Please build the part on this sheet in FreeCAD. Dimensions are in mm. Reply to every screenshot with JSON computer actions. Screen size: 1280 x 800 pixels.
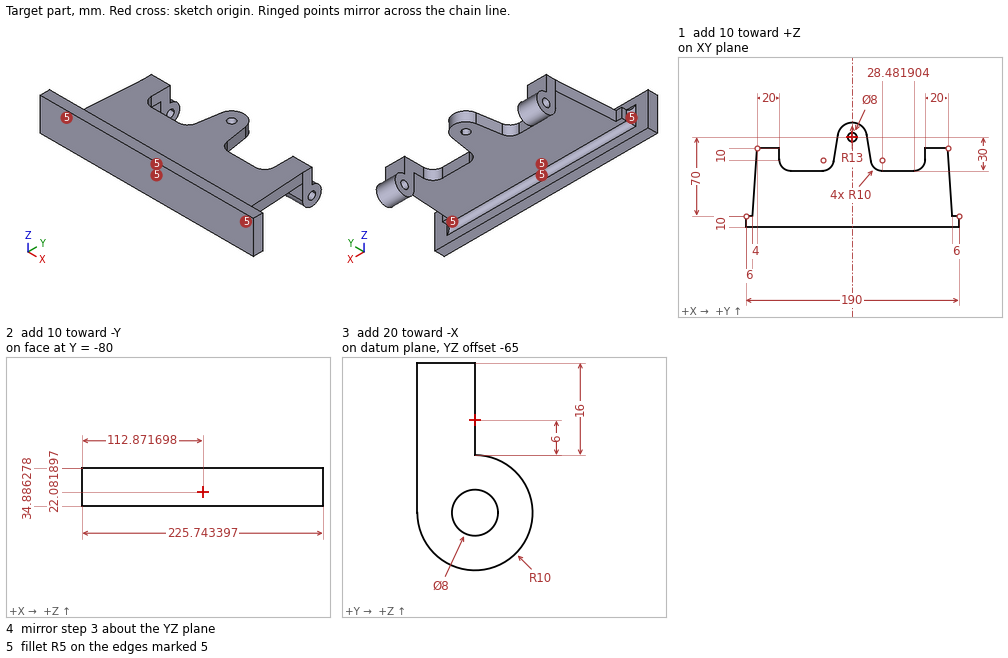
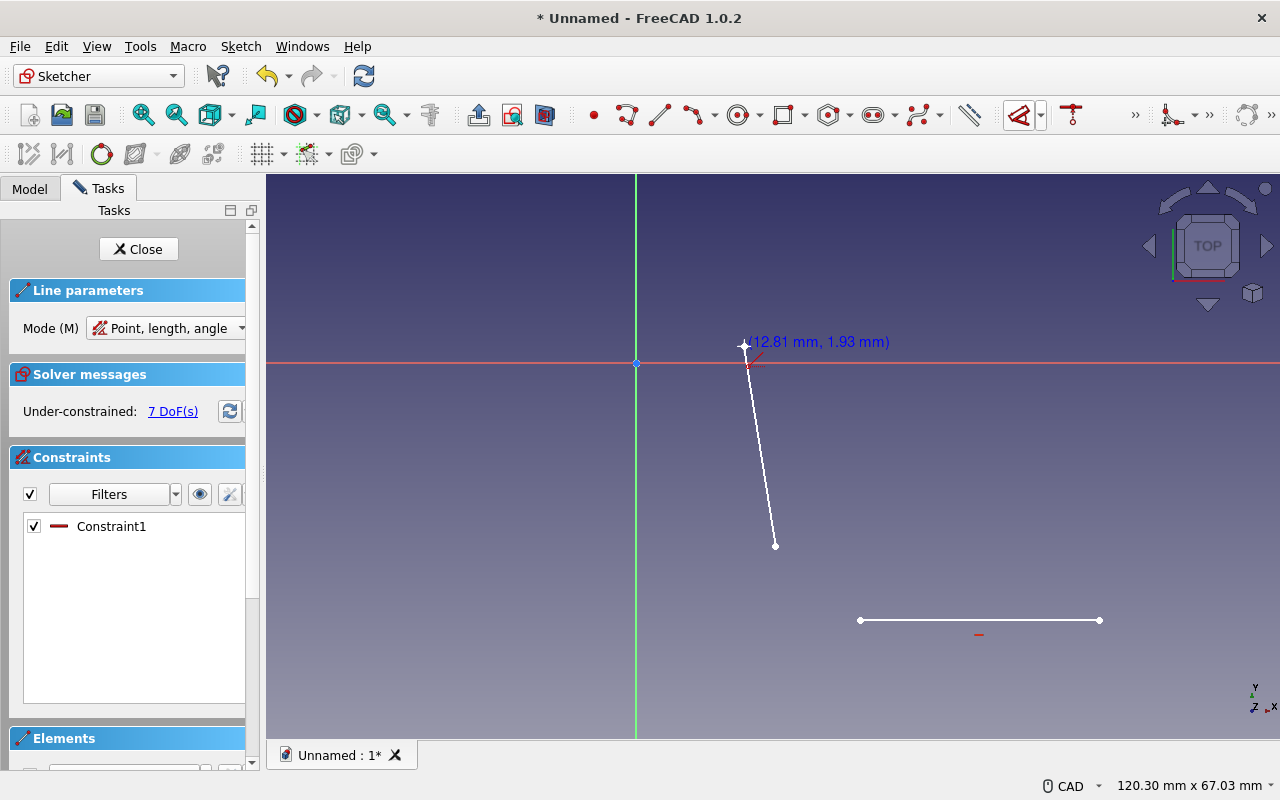
{"action": "left_click", "coordinate": [528, 346]}
{"action": "left_click", "coordinate": [496, 545]}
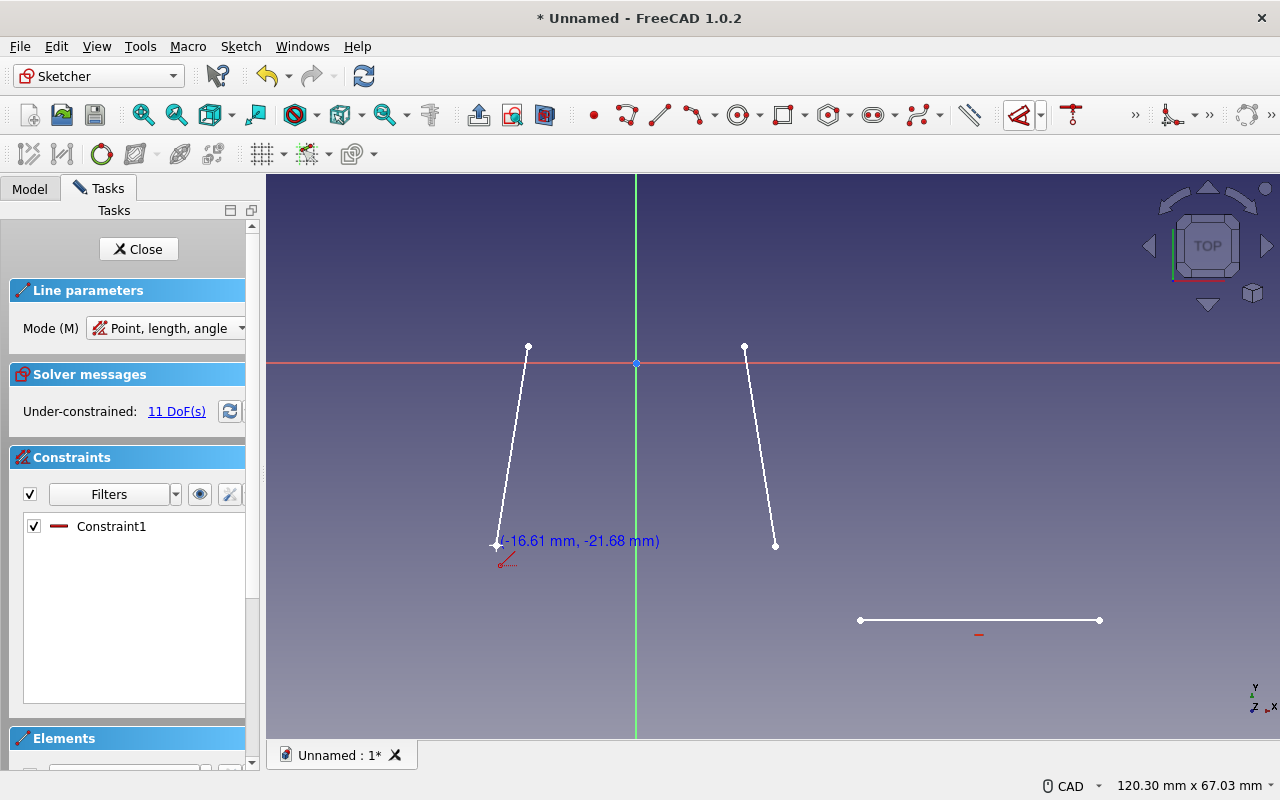
{"action": "left_click", "coordinate": [413, 616]}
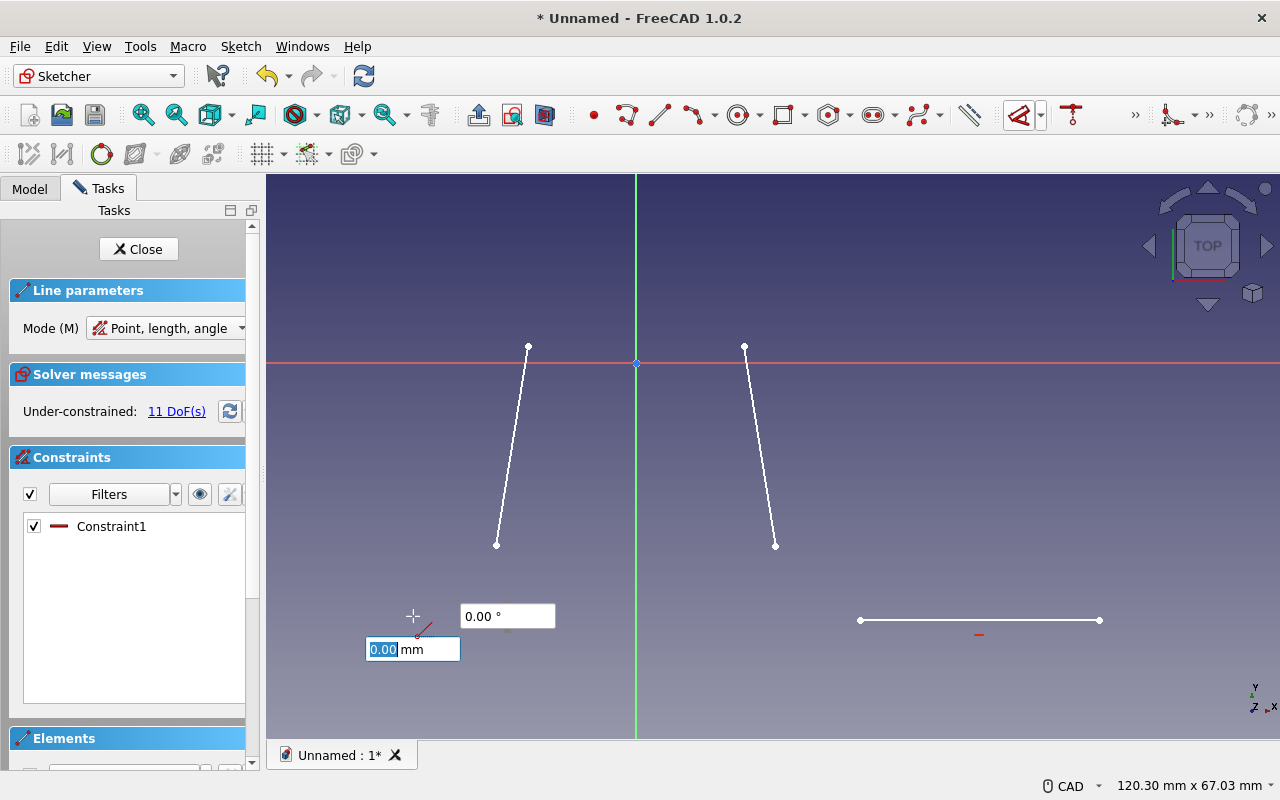
{"action": "scroll", "coordinate": [744, 346], "scroll_direction": "down", "scroll_amount": 5}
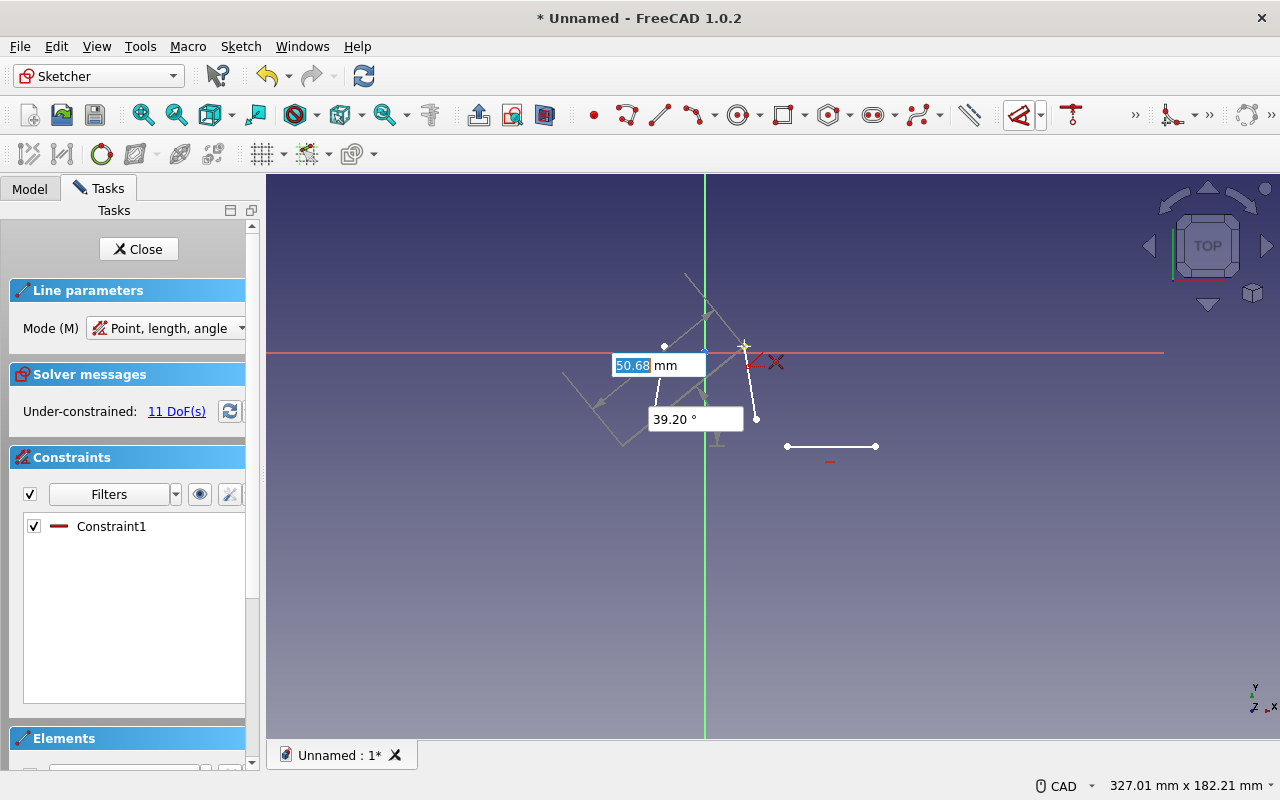
{"action": "left_click", "coordinate": [534, 446]}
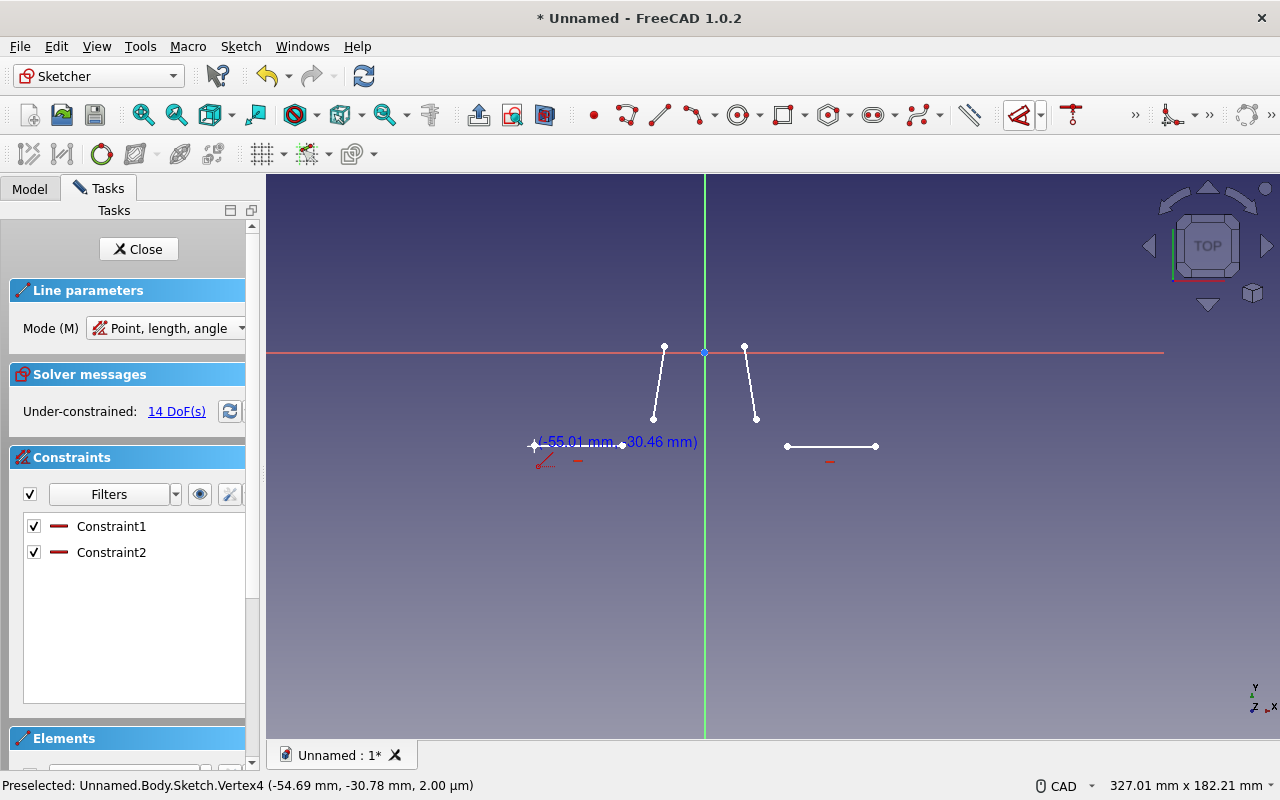
{"action": "left_click", "coordinate": [627, 116]}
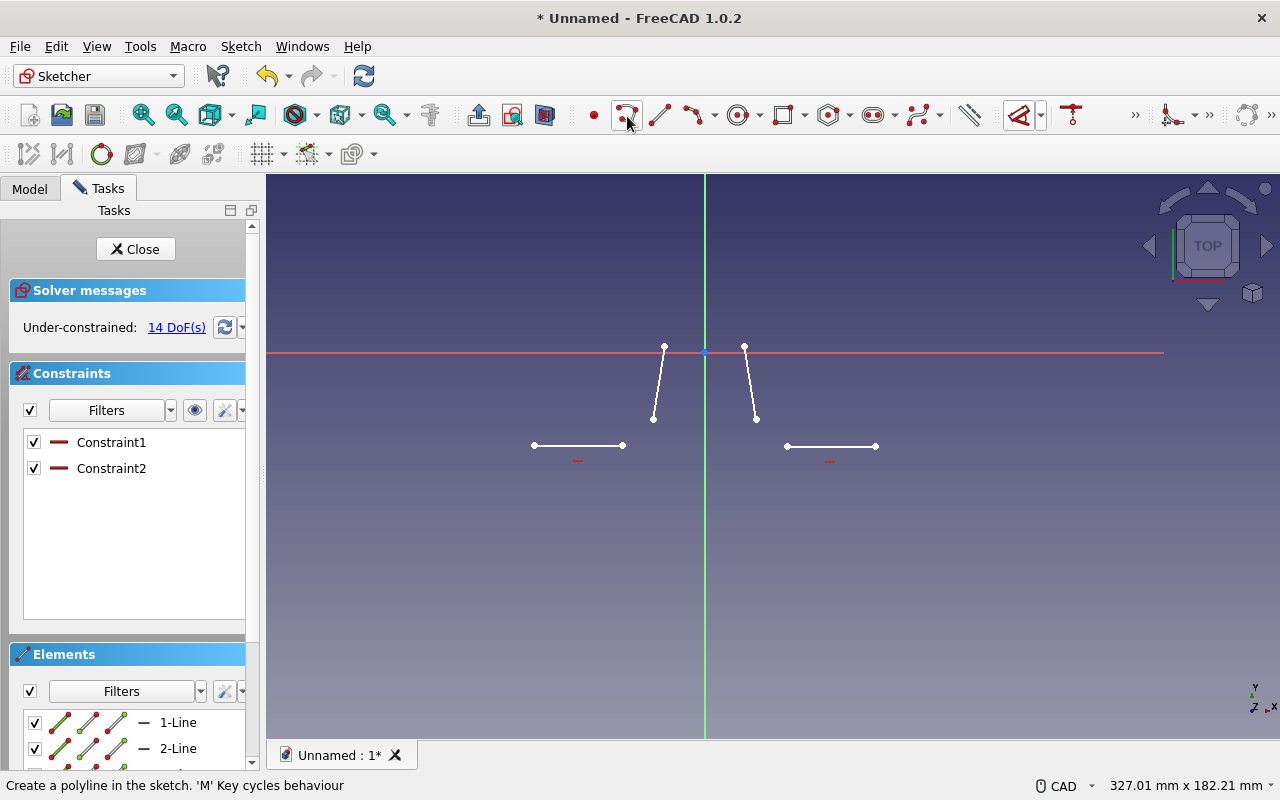
{"action": "left_click", "coordinate": [503, 415]}
{"action": "left_click", "coordinate": [503, 384]}
{"action": "left_click", "coordinate": [441, 384]}
{"action": "left_click", "coordinate": [429, 570]}
{"action": "left_click", "coordinate": [410, 570]}
{"action": "left_click", "coordinate": [410, 601]}
{"action": "left_click", "coordinate": [999, 601]}
{"action": "left_click", "coordinate": [999, 570]}
{"action": "left_click", "coordinate": [981, 570]}
{"action": "left_click", "coordinate": [968, 384]}
{"action": "left_click", "coordinate": [906, 384]}
{"action": "left_click", "coordinate": [906, 415]}
{"action": "right_click", "coordinate": [906, 415]}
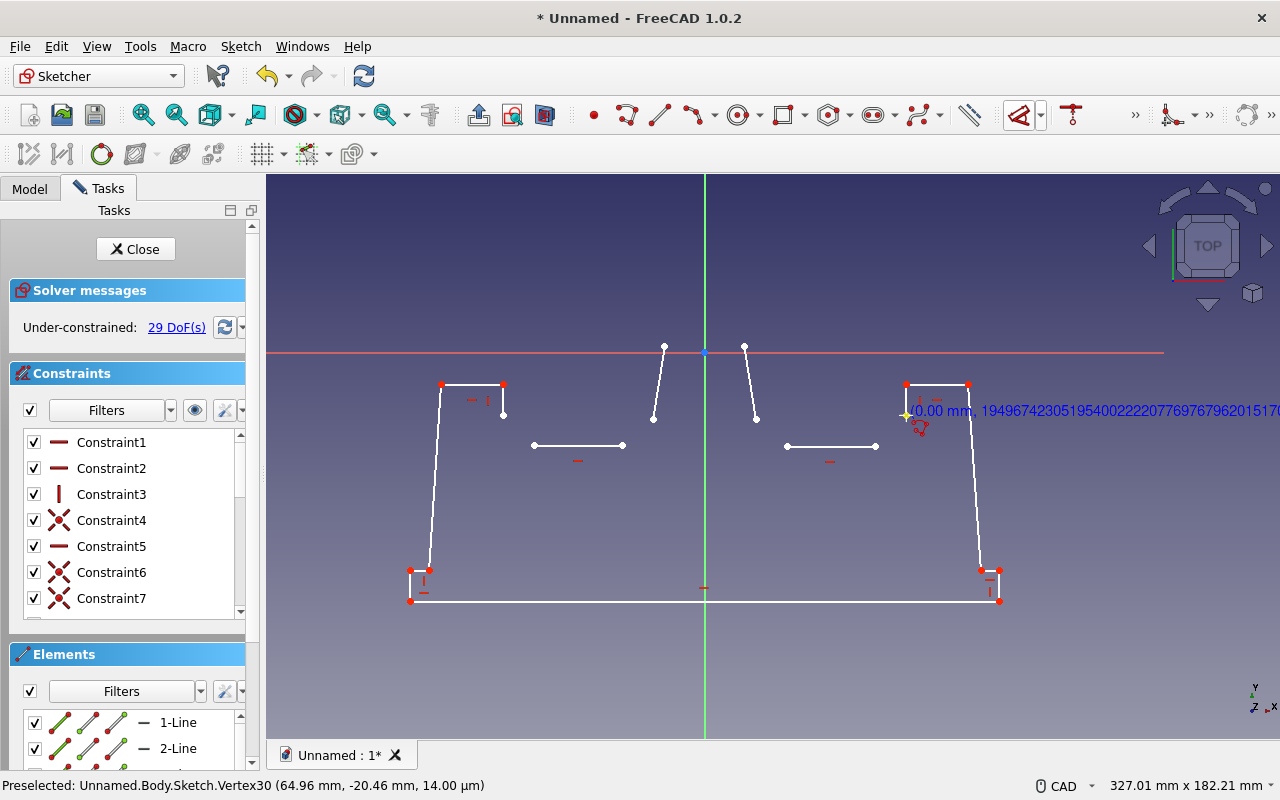
{"action": "left_click", "coordinate": [692, 116]}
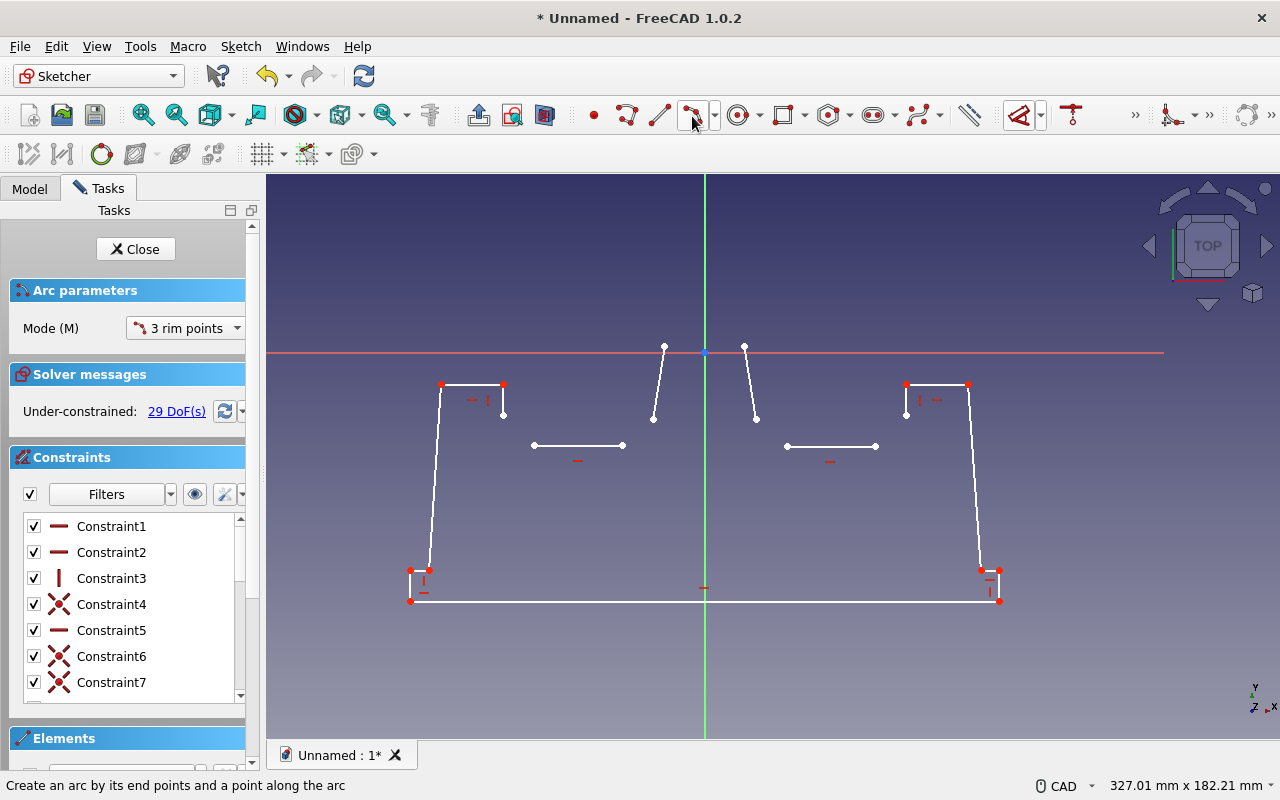
{"action": "left_click", "coordinate": [787, 447]}
{"action": "left_click", "coordinate": [756, 420]}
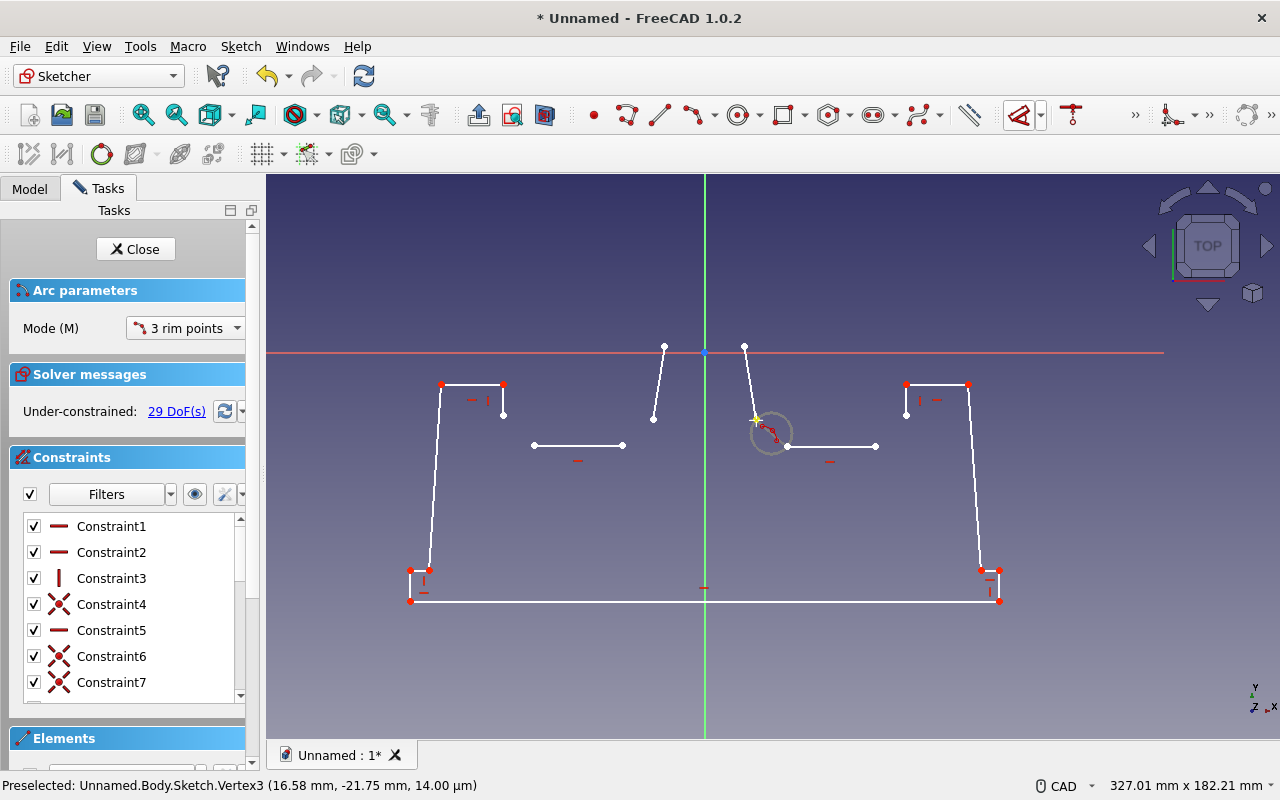
{"action": "scroll", "coordinate": [767, 438], "scroll_direction": "up", "scroll_amount": 4}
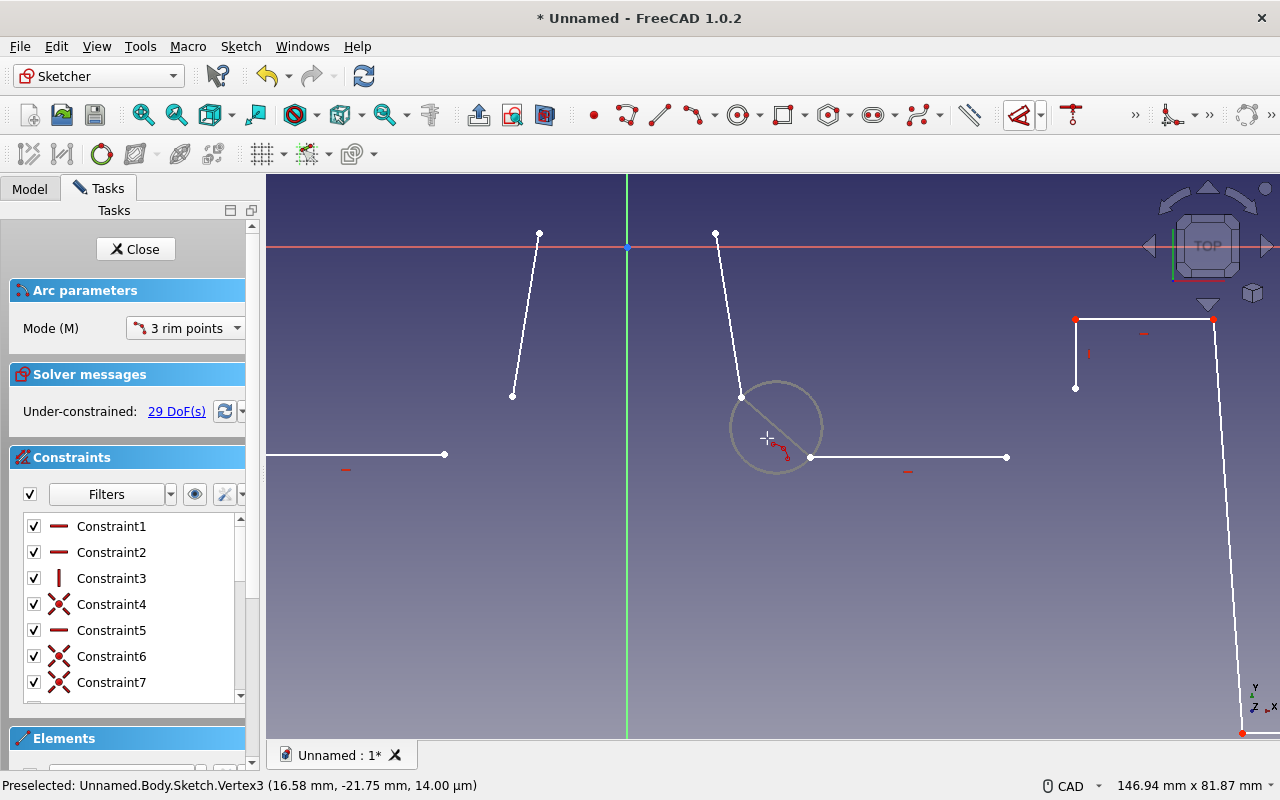
{"action": "left_click", "coordinate": [766, 438]}